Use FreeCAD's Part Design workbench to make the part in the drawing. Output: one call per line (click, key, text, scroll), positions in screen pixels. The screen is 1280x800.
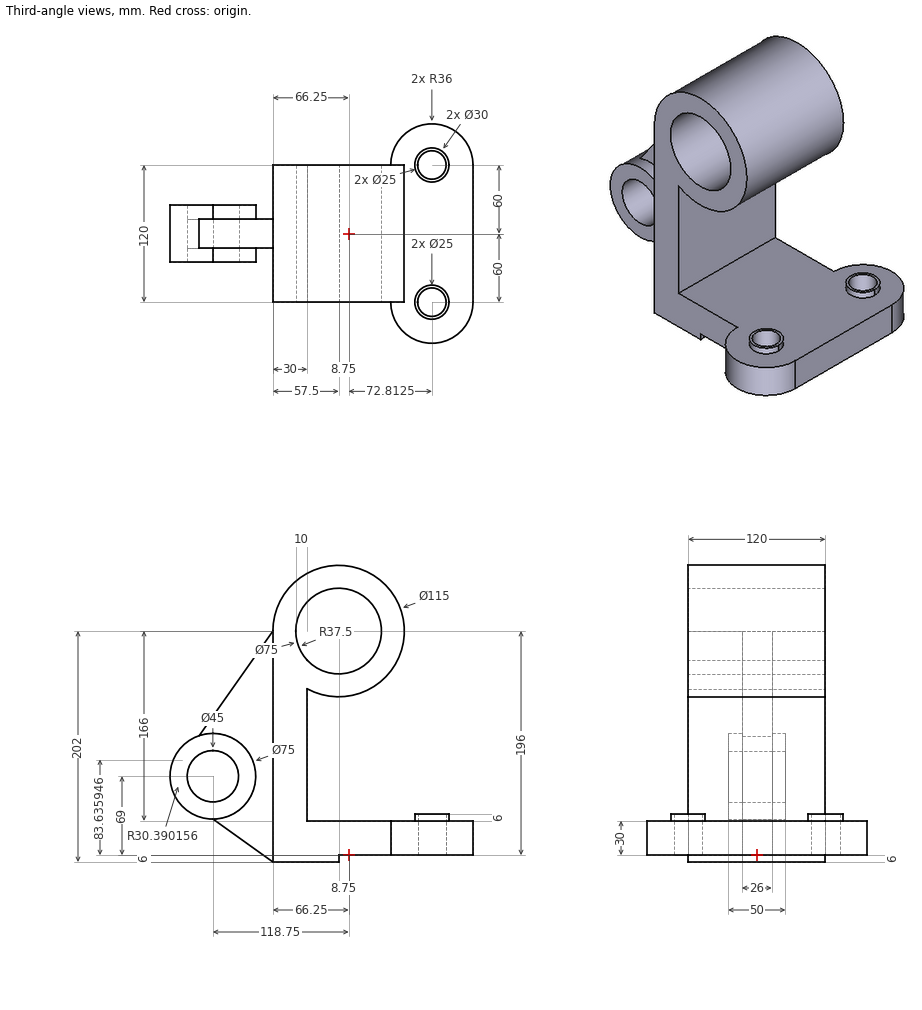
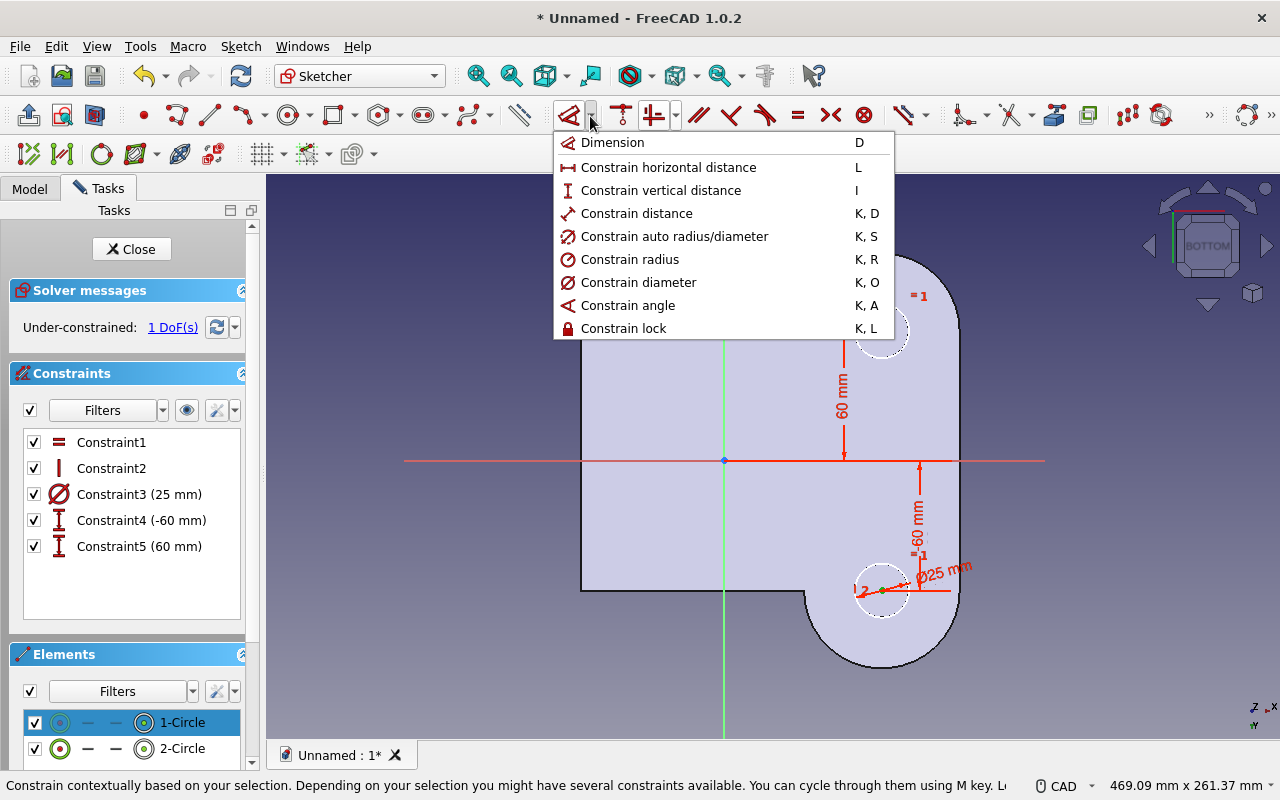
click(724, 168)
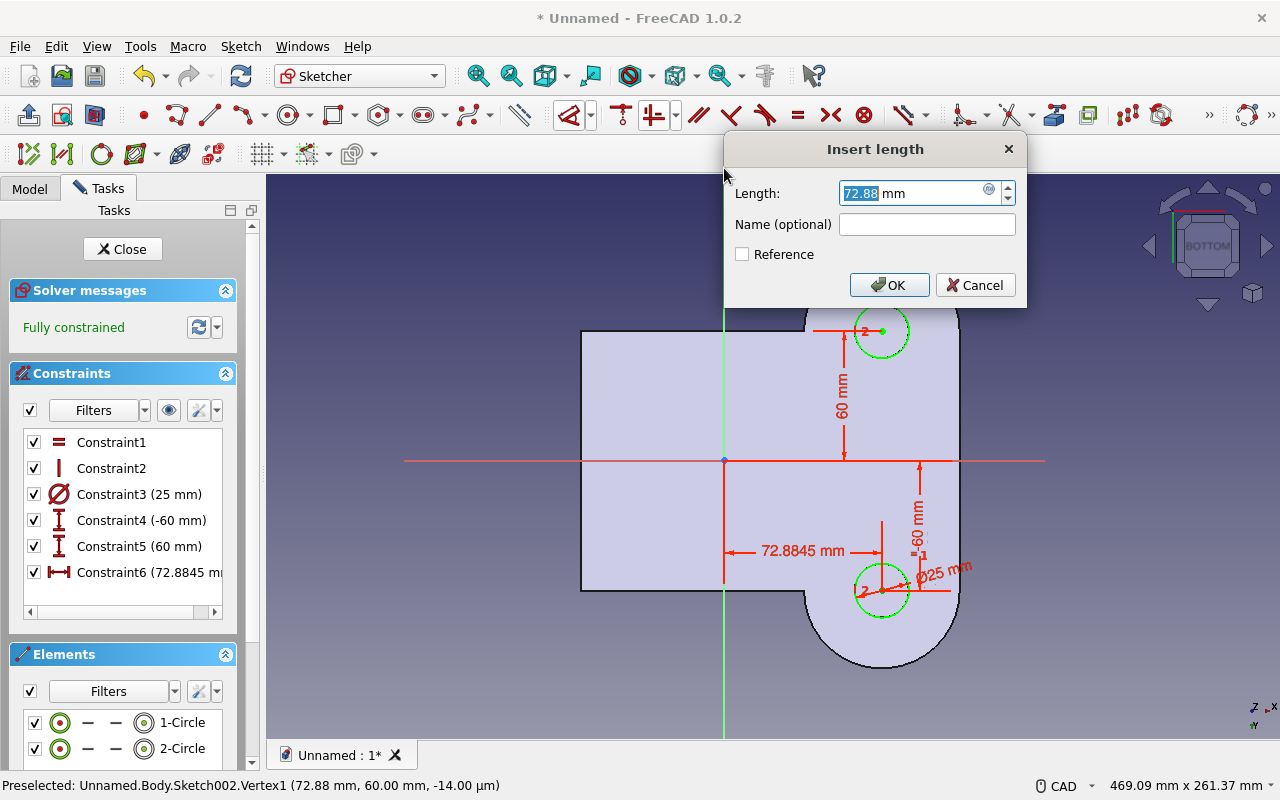
text(72.8125)
key(Return)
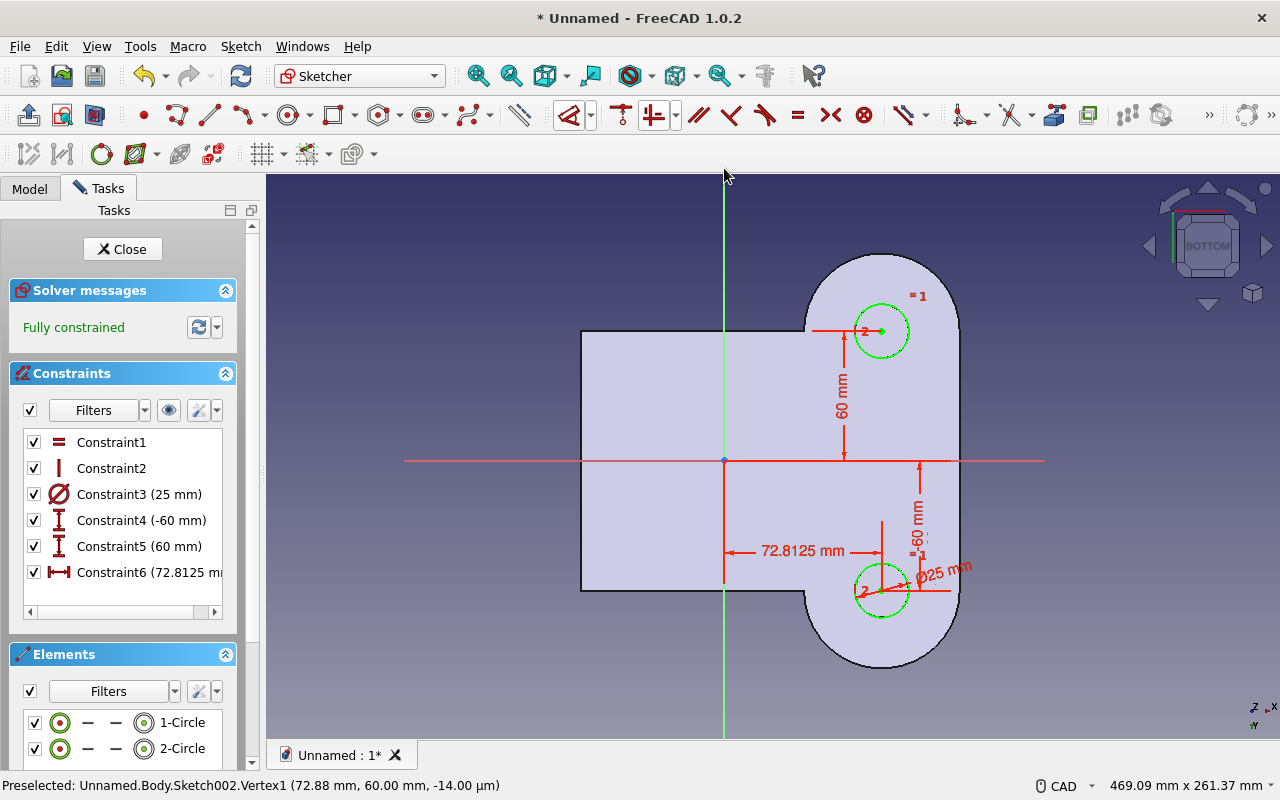
click(123, 249)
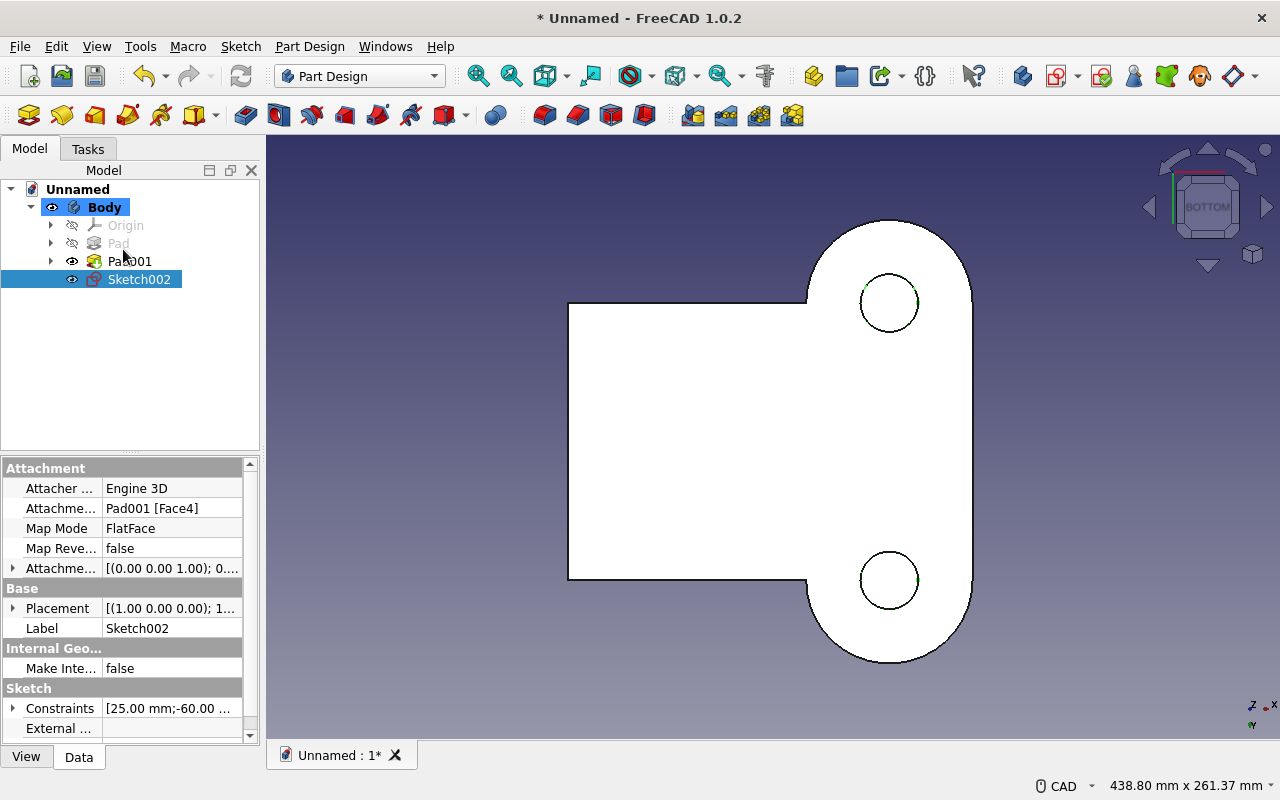
click(246, 116)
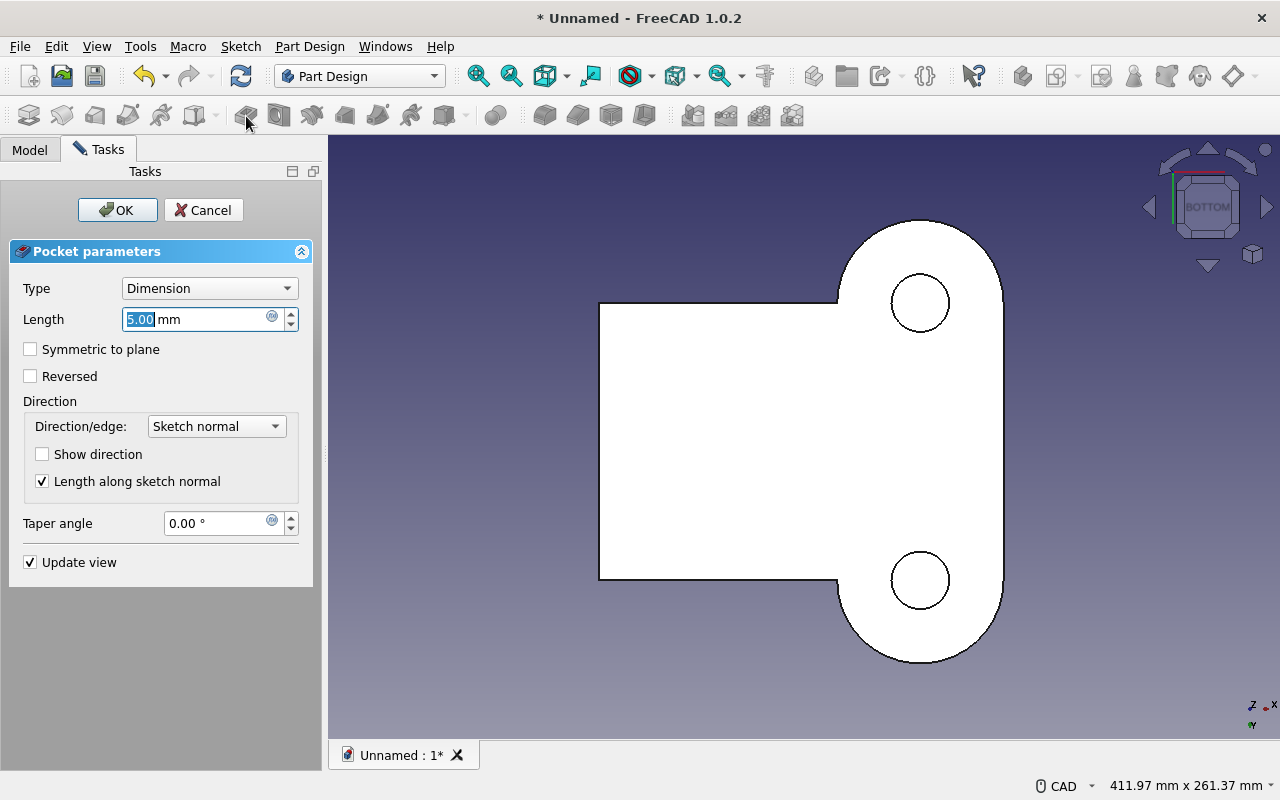
click(210, 288)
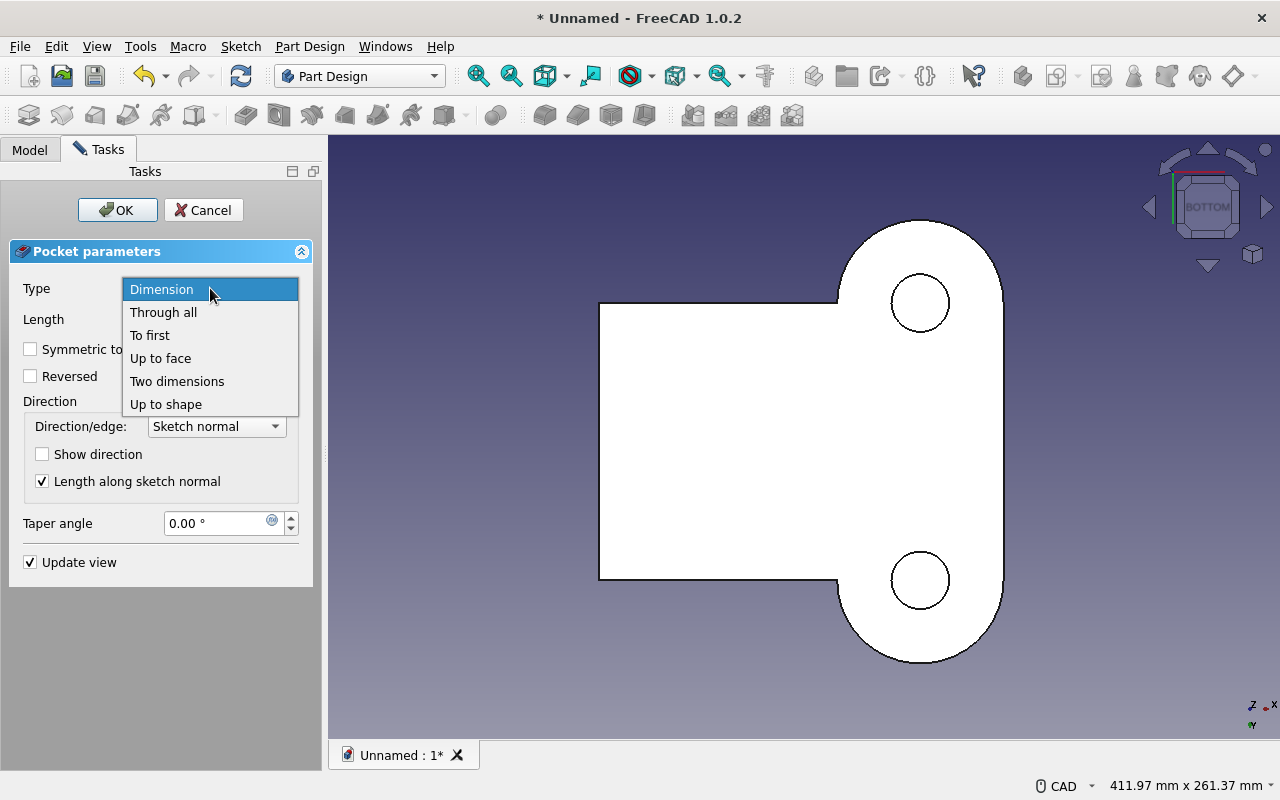
click(208, 312)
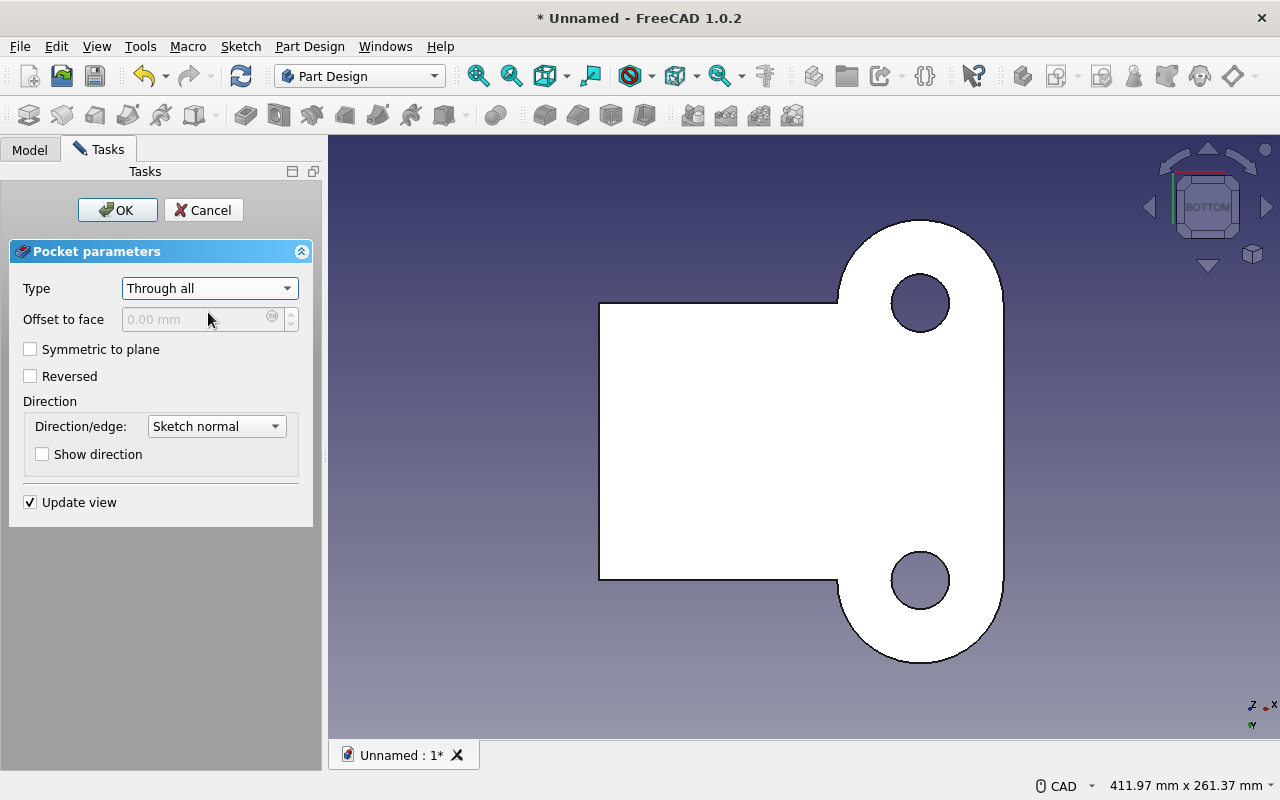
click(118, 210)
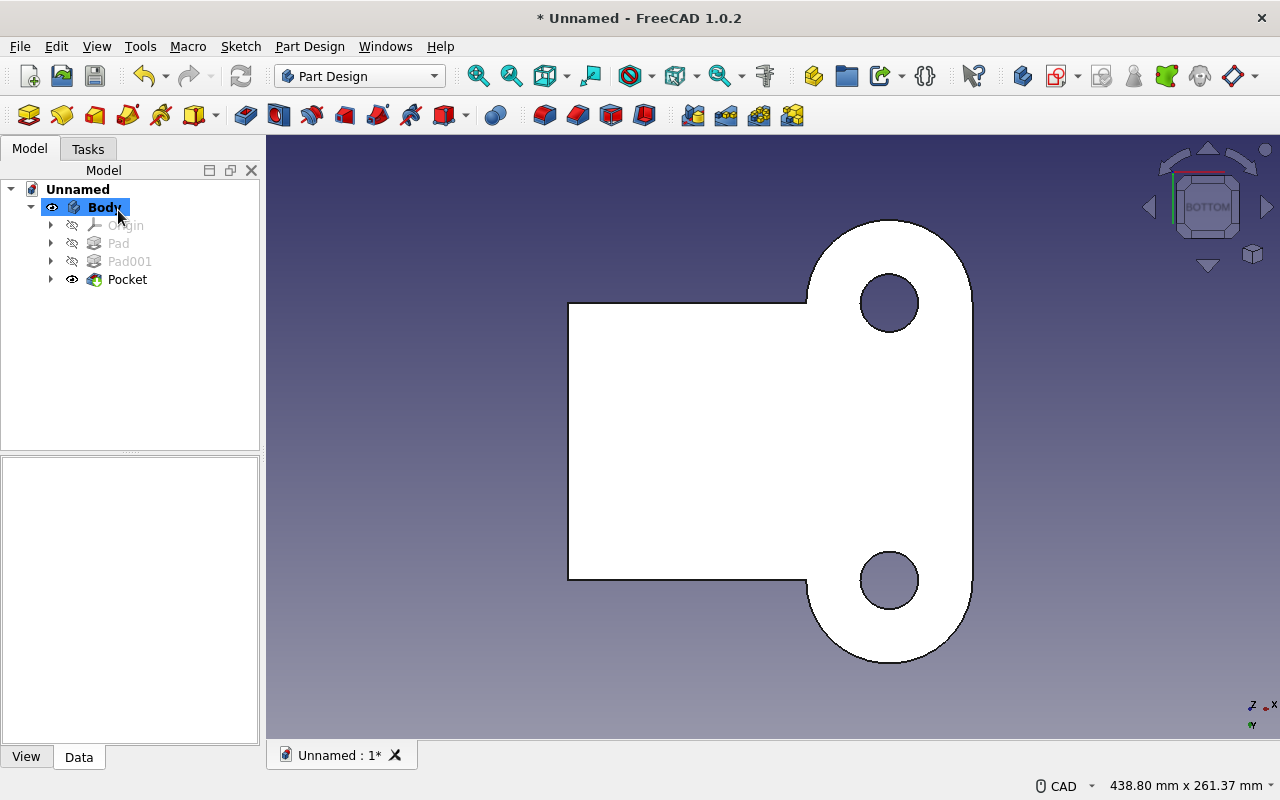
click(1056, 76)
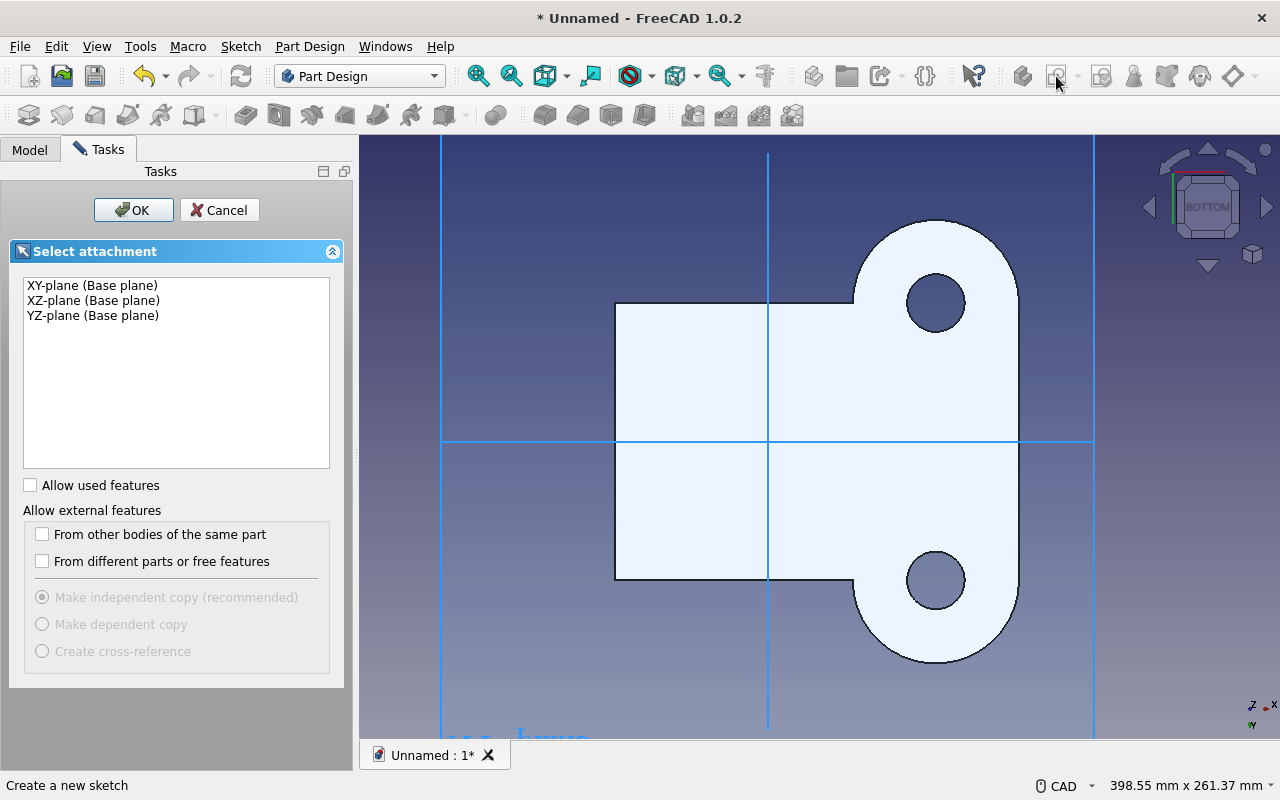
click(84, 286)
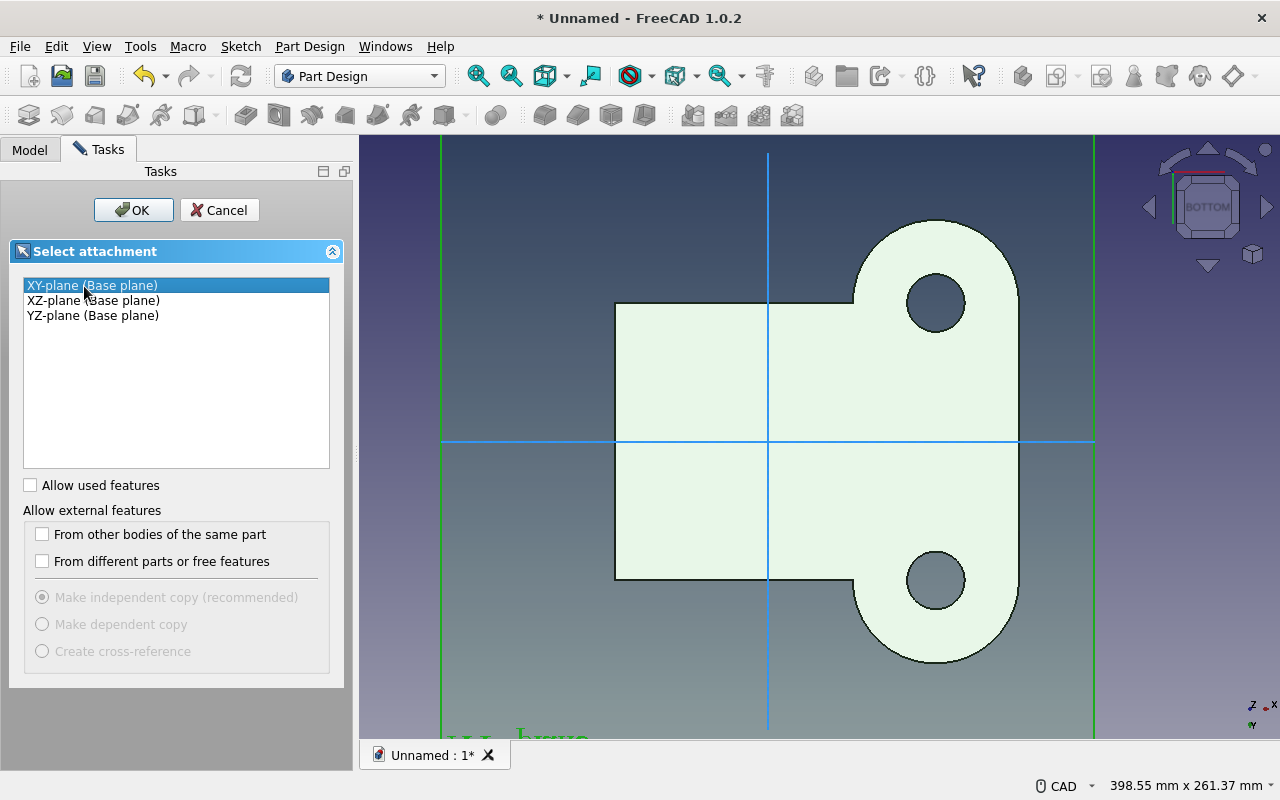
click(134, 210)